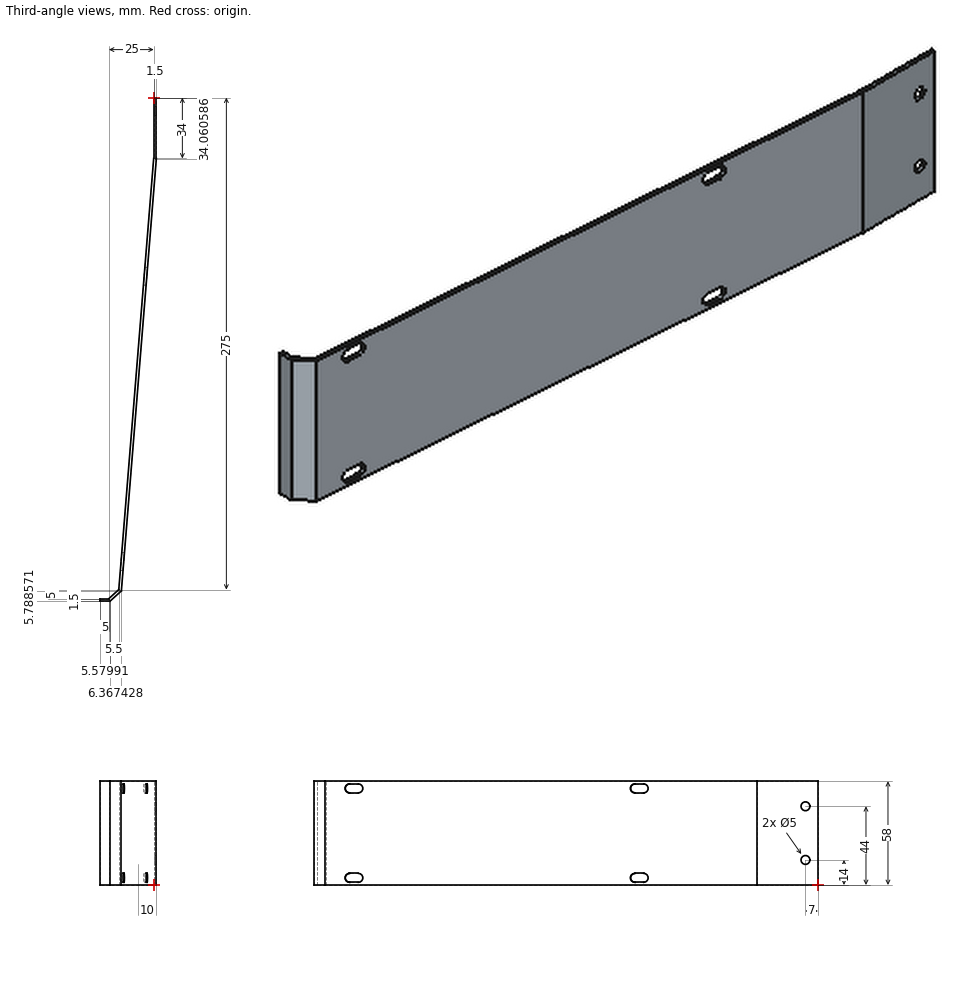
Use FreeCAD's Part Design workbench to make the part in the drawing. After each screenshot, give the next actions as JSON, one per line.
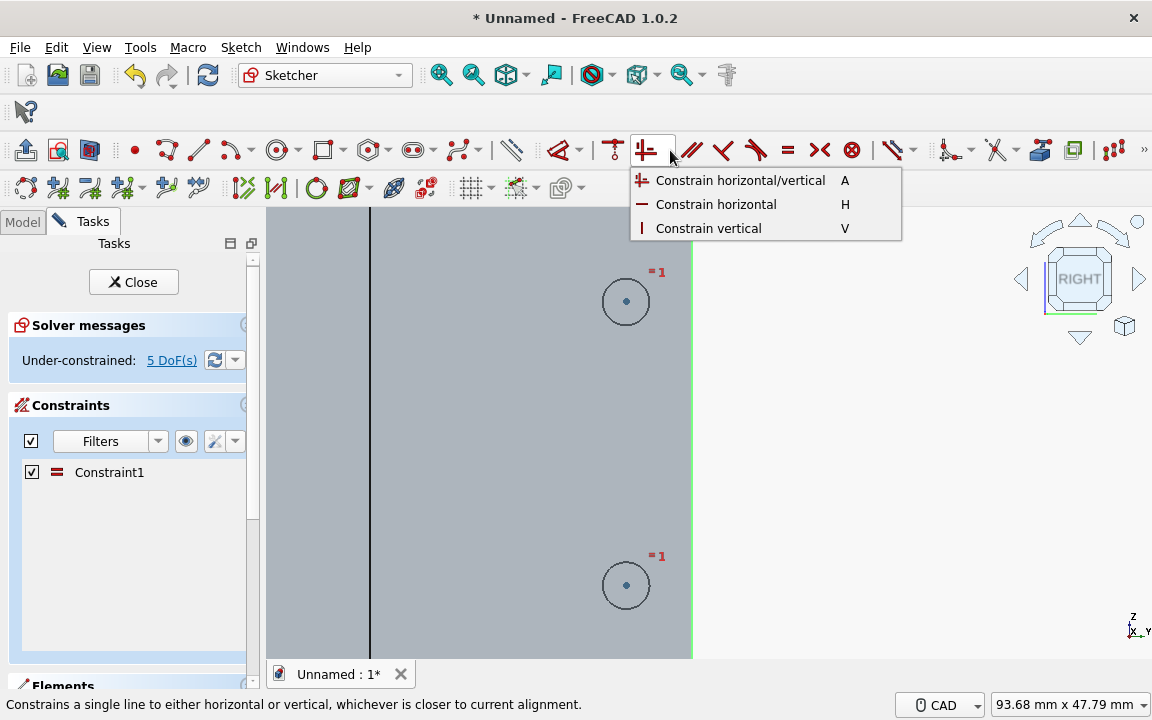
{"action": "left_click", "coordinate": [766, 228]}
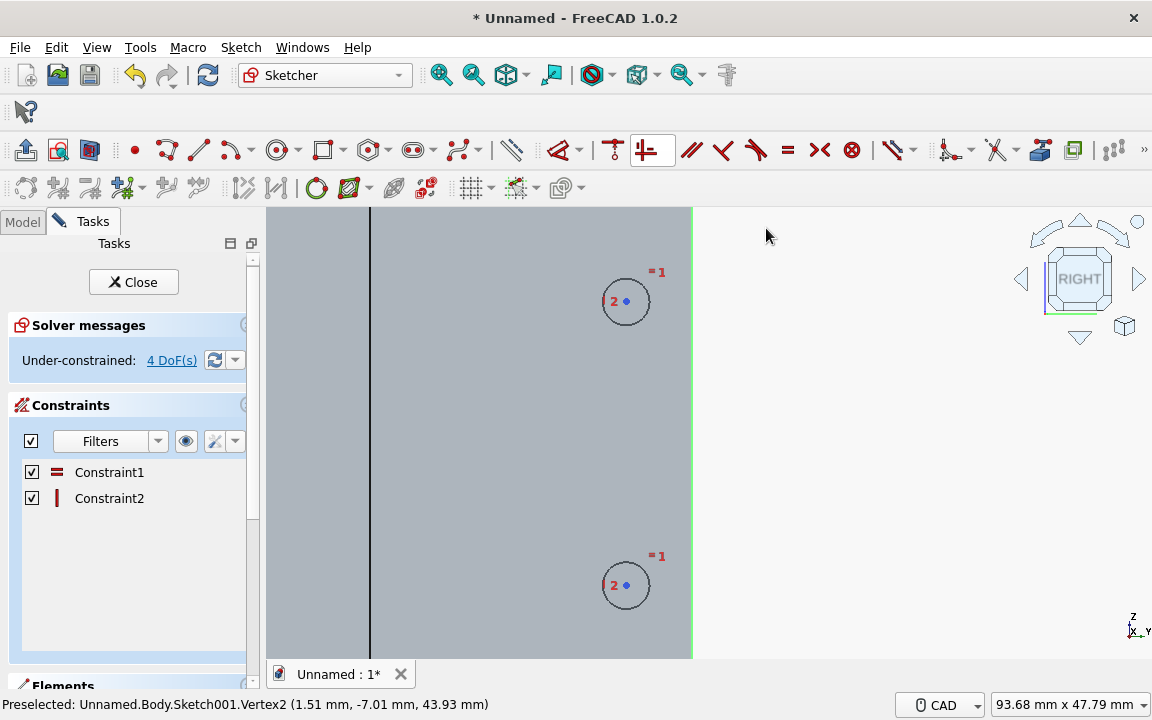
{"action": "left_click", "coordinate": [558, 150]}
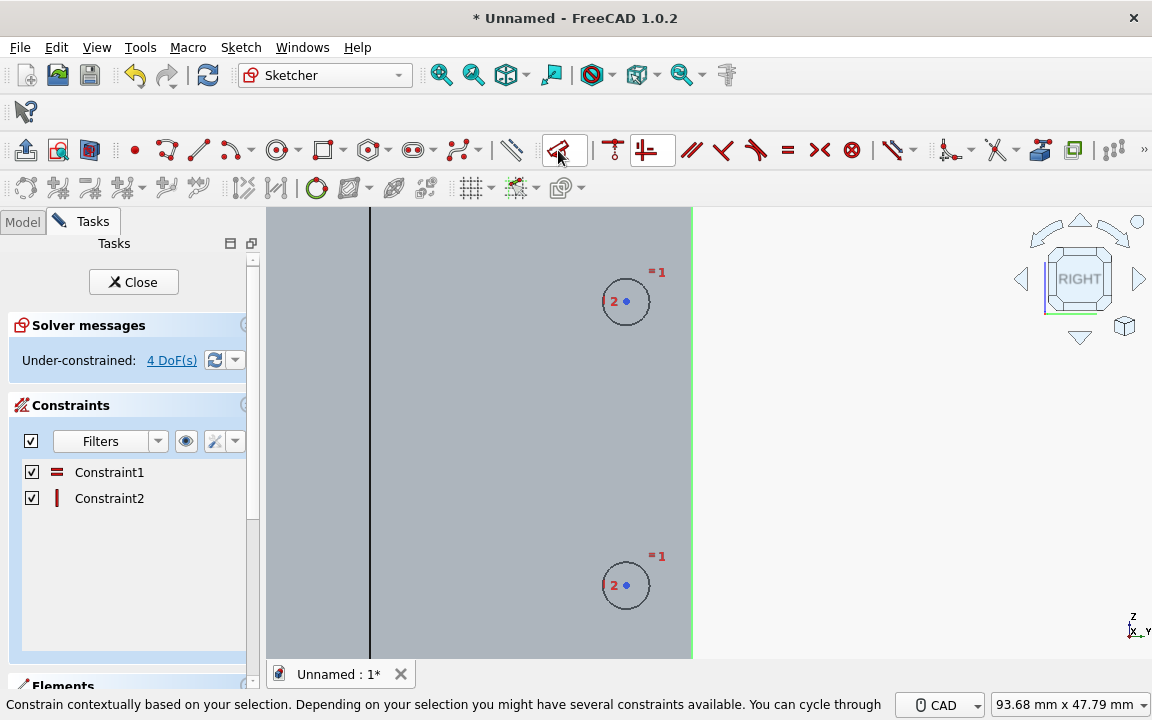
{"action": "left_click", "coordinate": [643, 569]}
{"action": "left_click", "coordinate": [666, 546]}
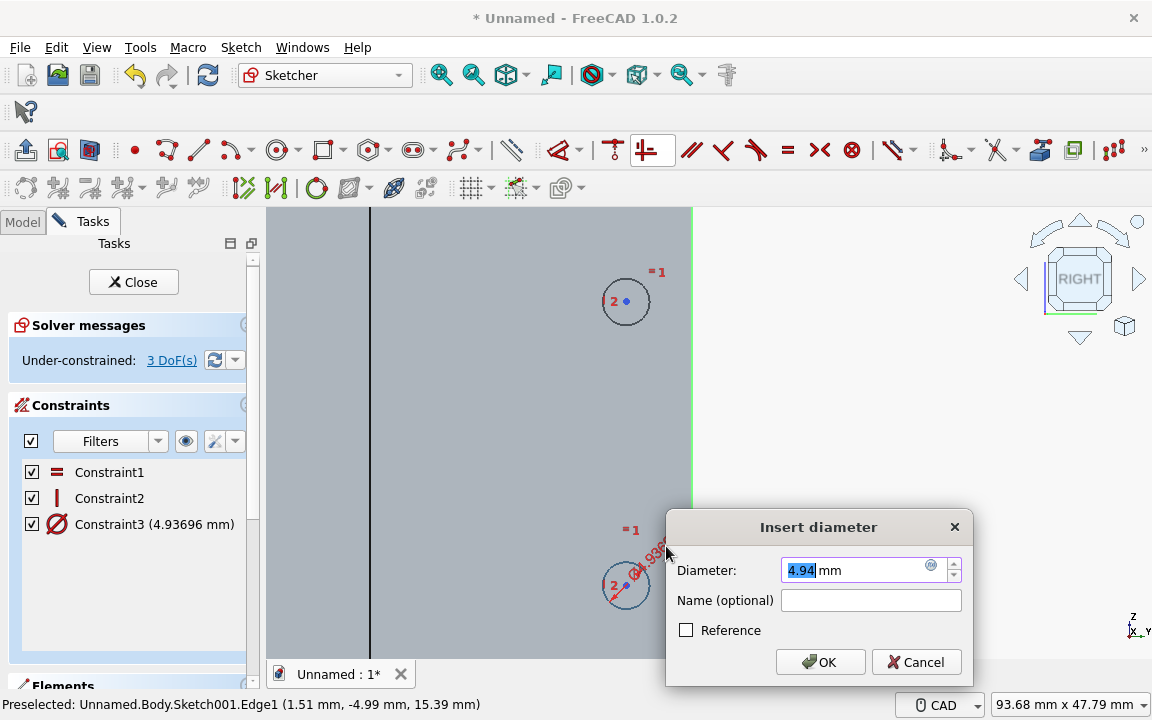
{"action": "type", "text": "5"}
{"action": "key", "text": "Return"}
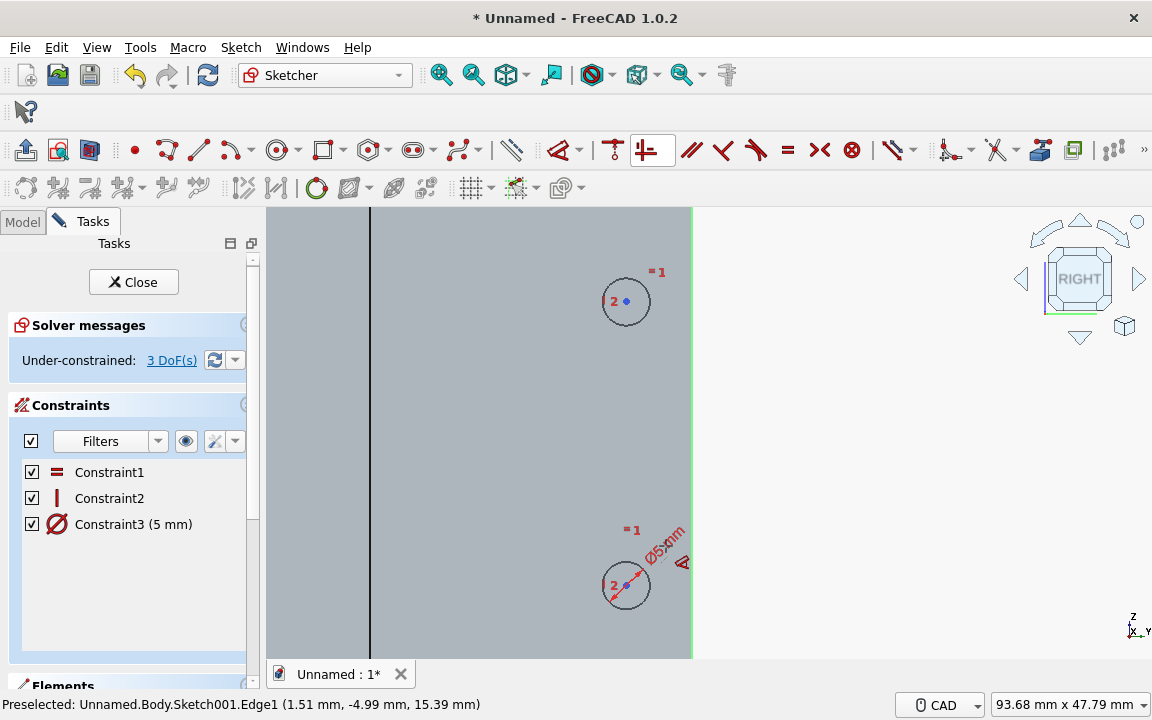
{"action": "left_click", "coordinate": [626, 586]}
{"action": "left_click", "coordinate": [659, 504]}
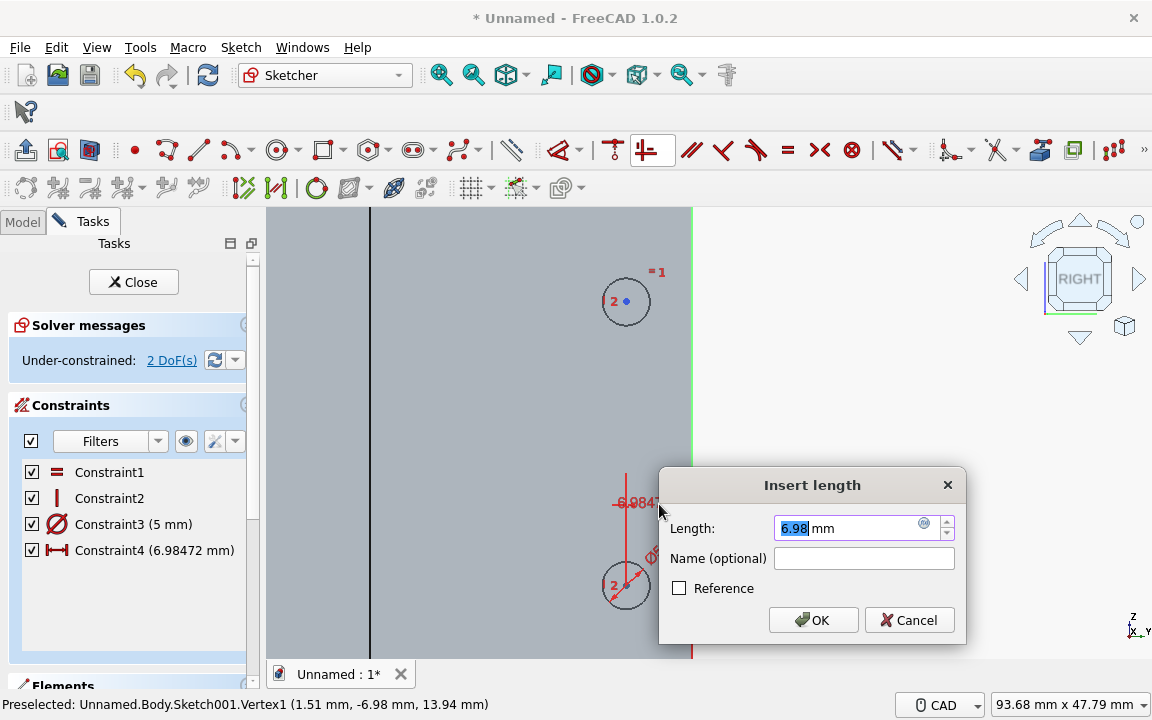
{"action": "type", "text": "7"}
{"action": "key", "text": "Return"}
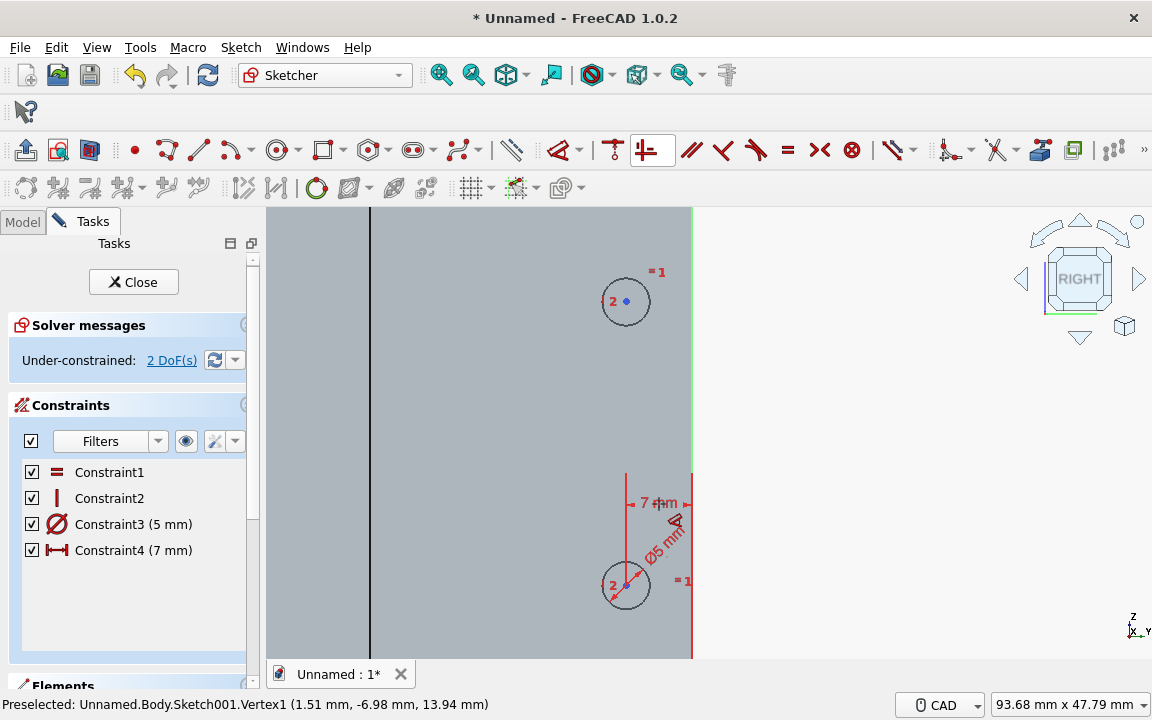
{"action": "left_click", "coordinate": [626, 586]}
{"action": "left_click", "coordinate": [726, 608]}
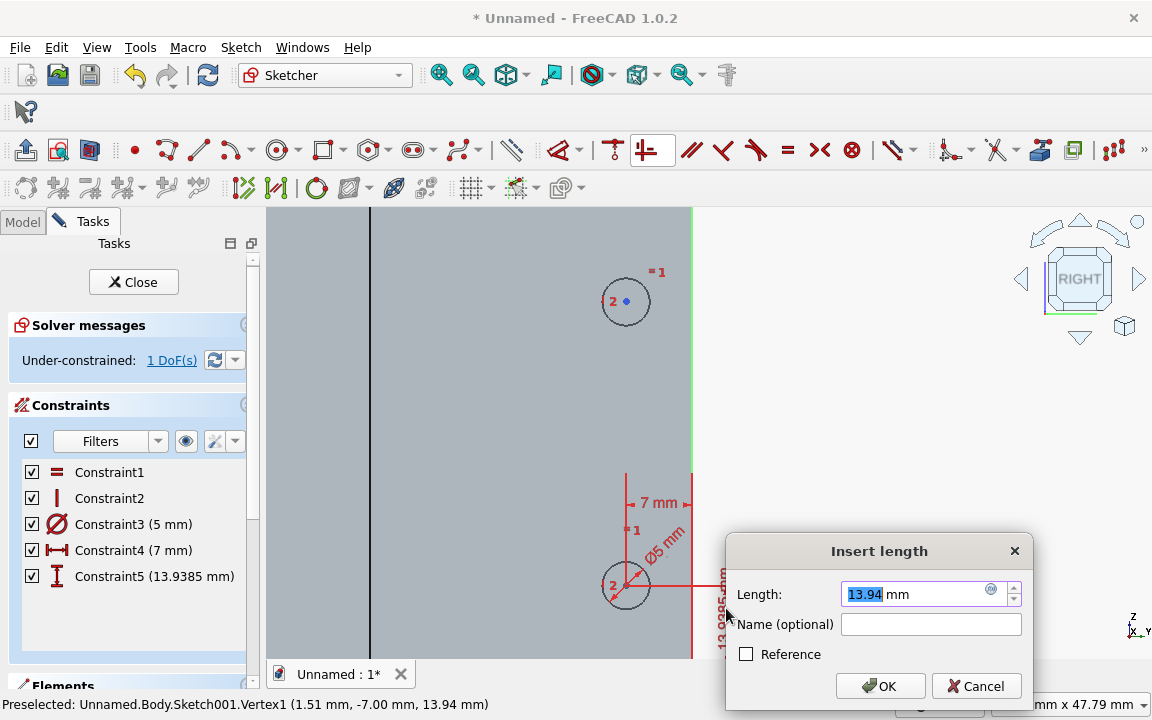
{"action": "type", "text": "14"}
{"action": "key", "text": "Return"}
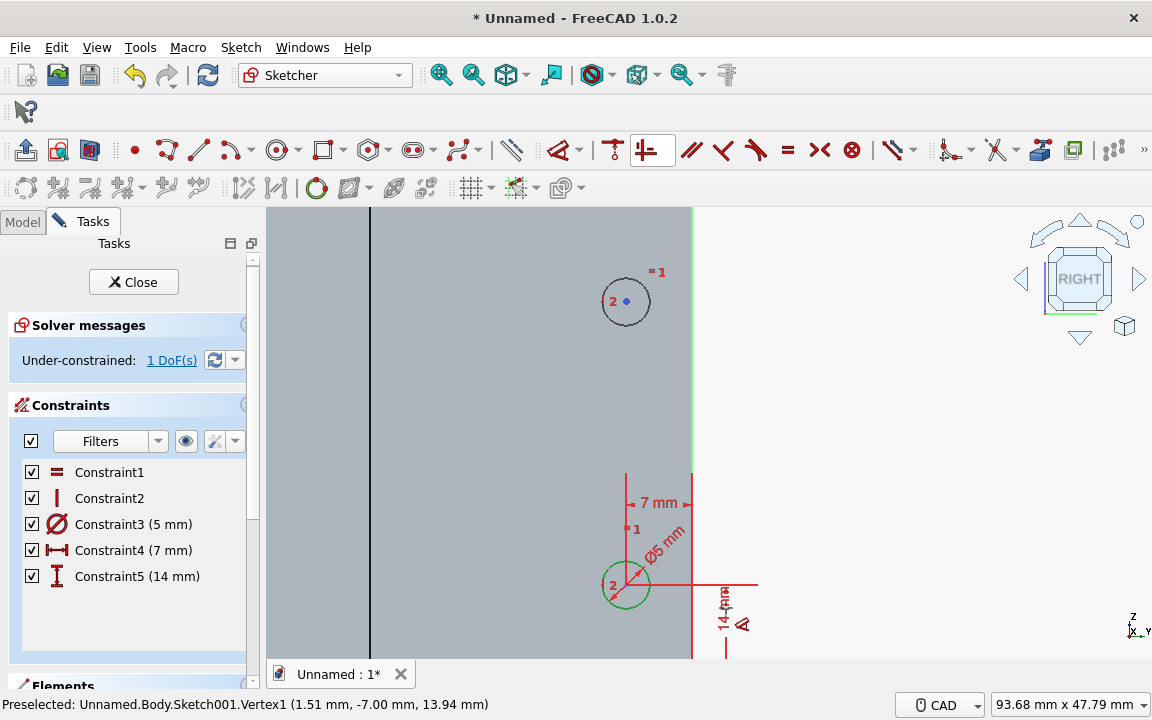
{"action": "left_click", "coordinate": [626, 302]}
{"action": "left_click", "coordinate": [726, 467]}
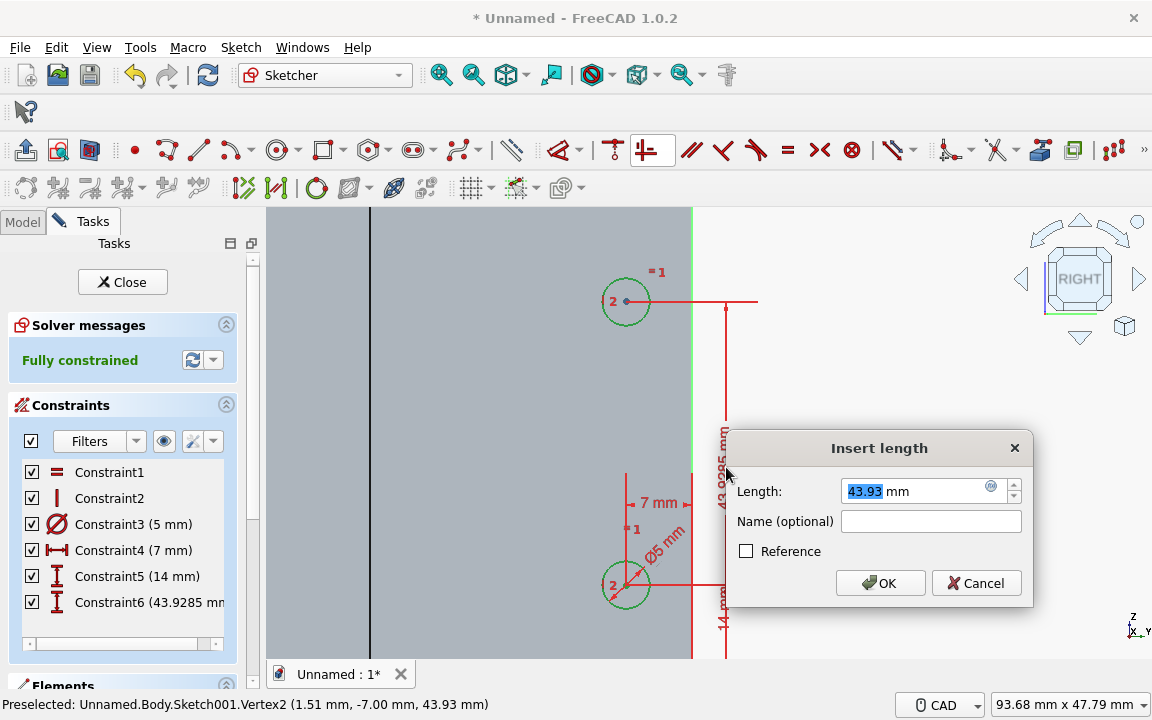
{"action": "type", "text": "44"}
{"action": "key", "text": "Return"}
{"action": "key", "text": "Escape"}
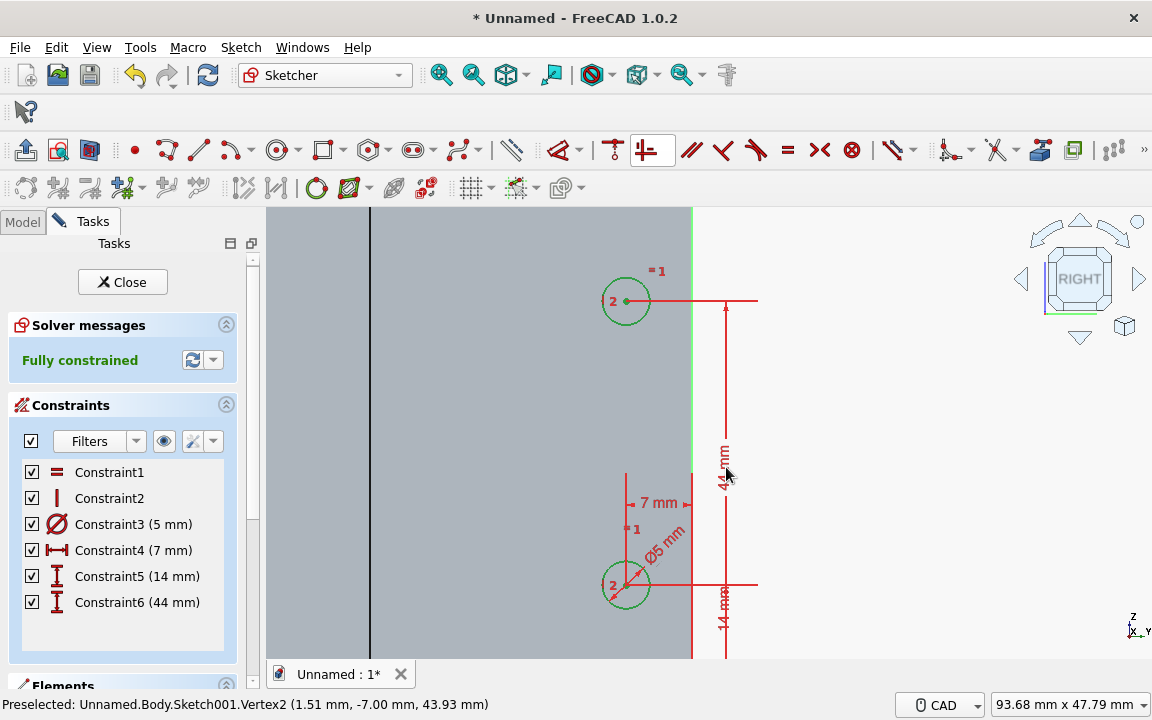
{"action": "left_click", "coordinate": [123, 282]}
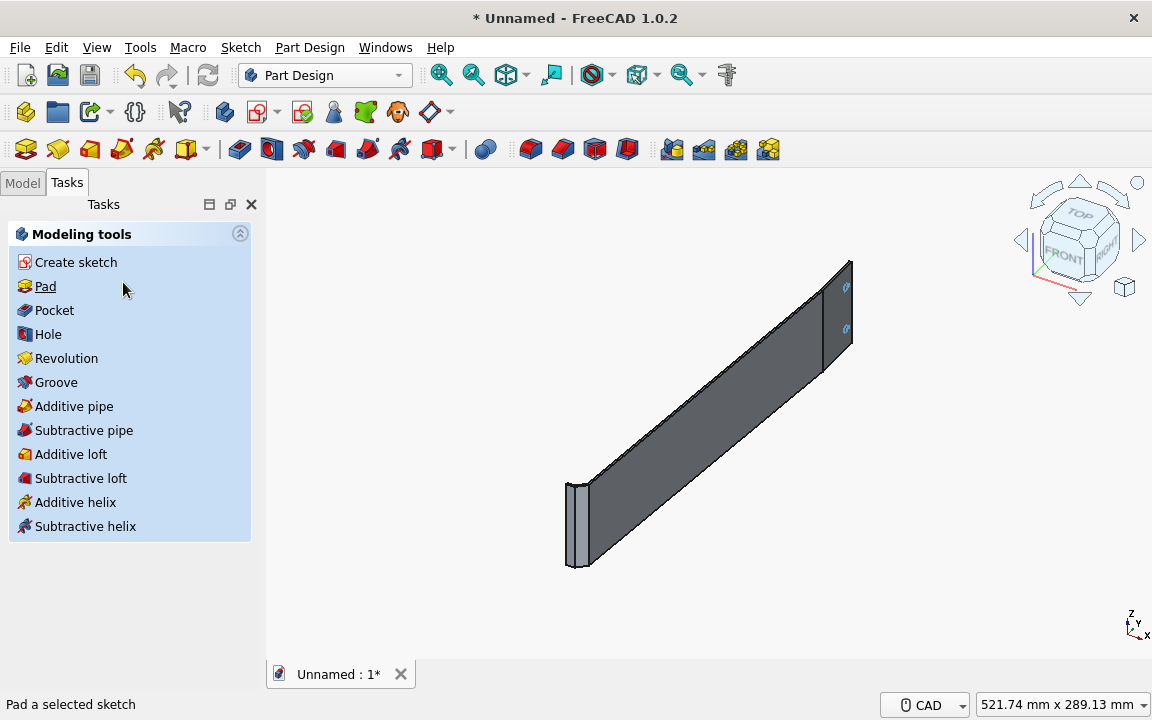
{"action": "left_click", "coordinate": [240, 150]}